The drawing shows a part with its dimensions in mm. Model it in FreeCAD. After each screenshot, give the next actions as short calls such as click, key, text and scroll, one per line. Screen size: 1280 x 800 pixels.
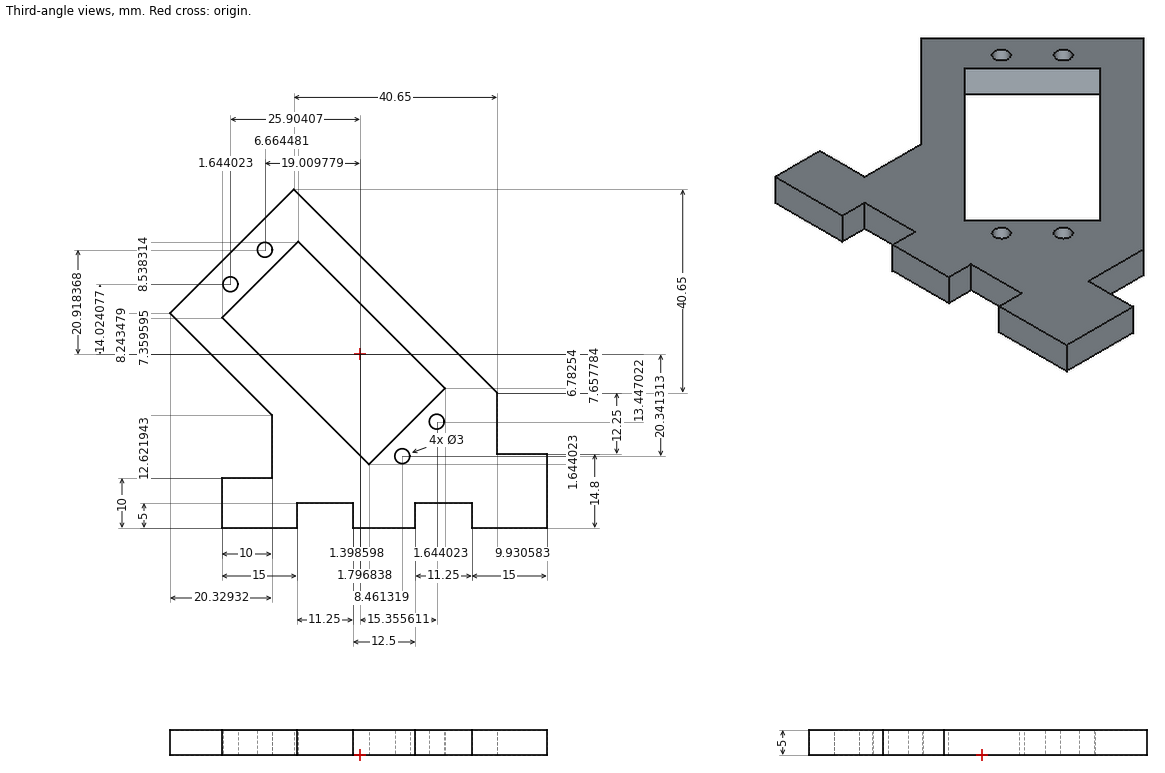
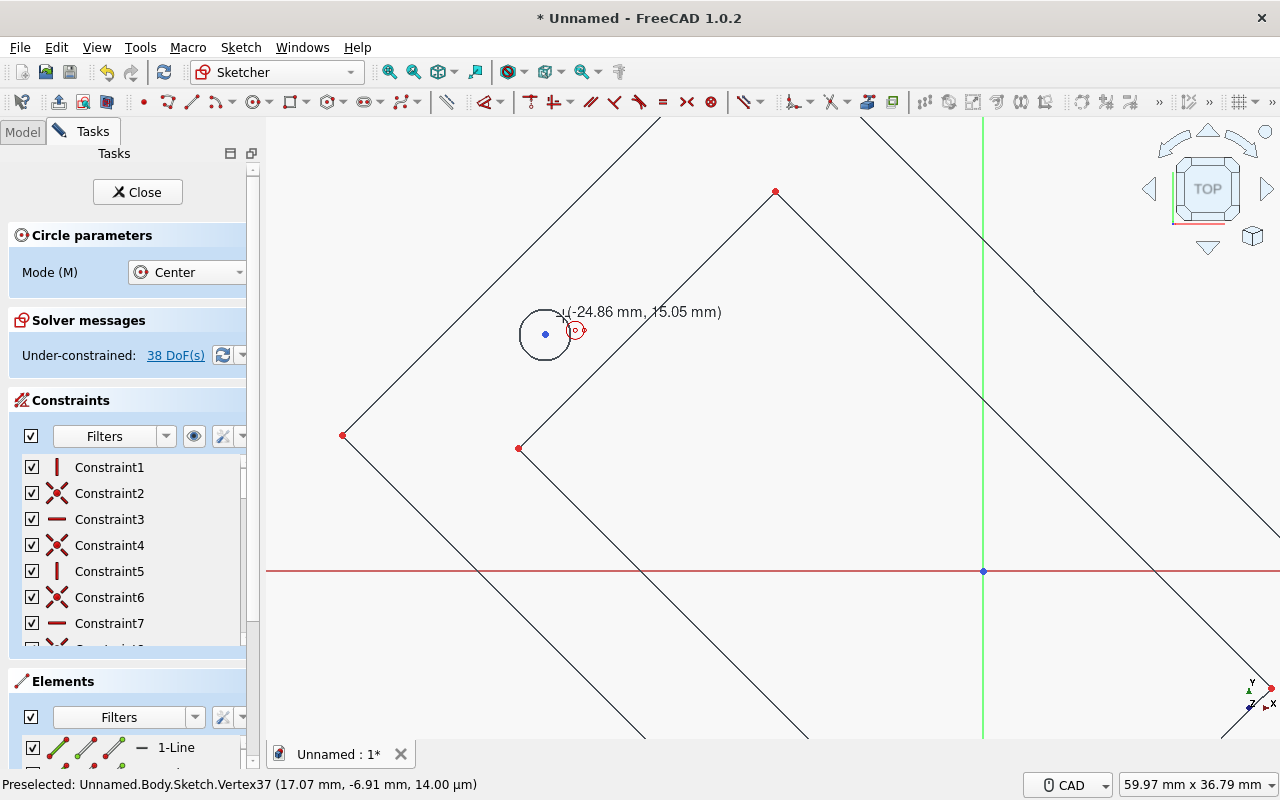
click(662, 218)
click(680, 200)
key(Escape)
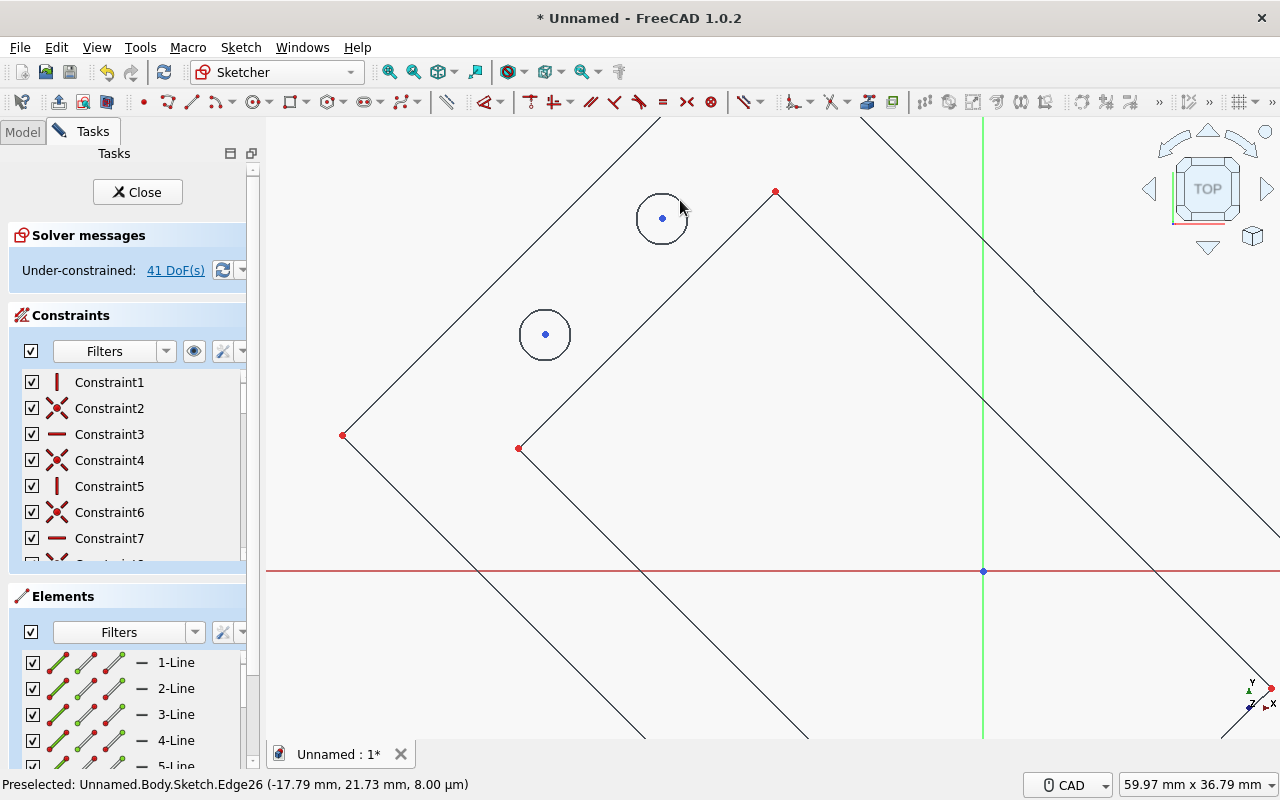
scroll(545, 336, down, 5)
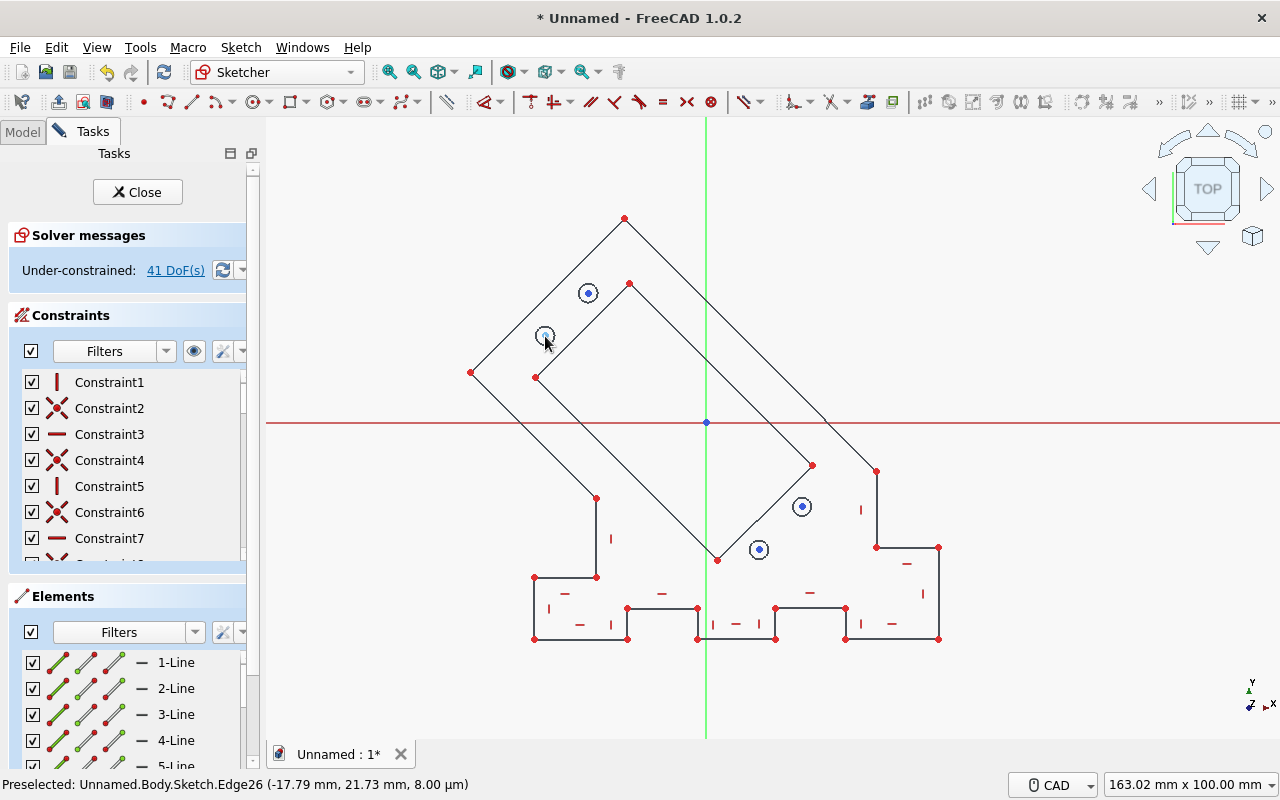
scroll(766, 543, up, 2)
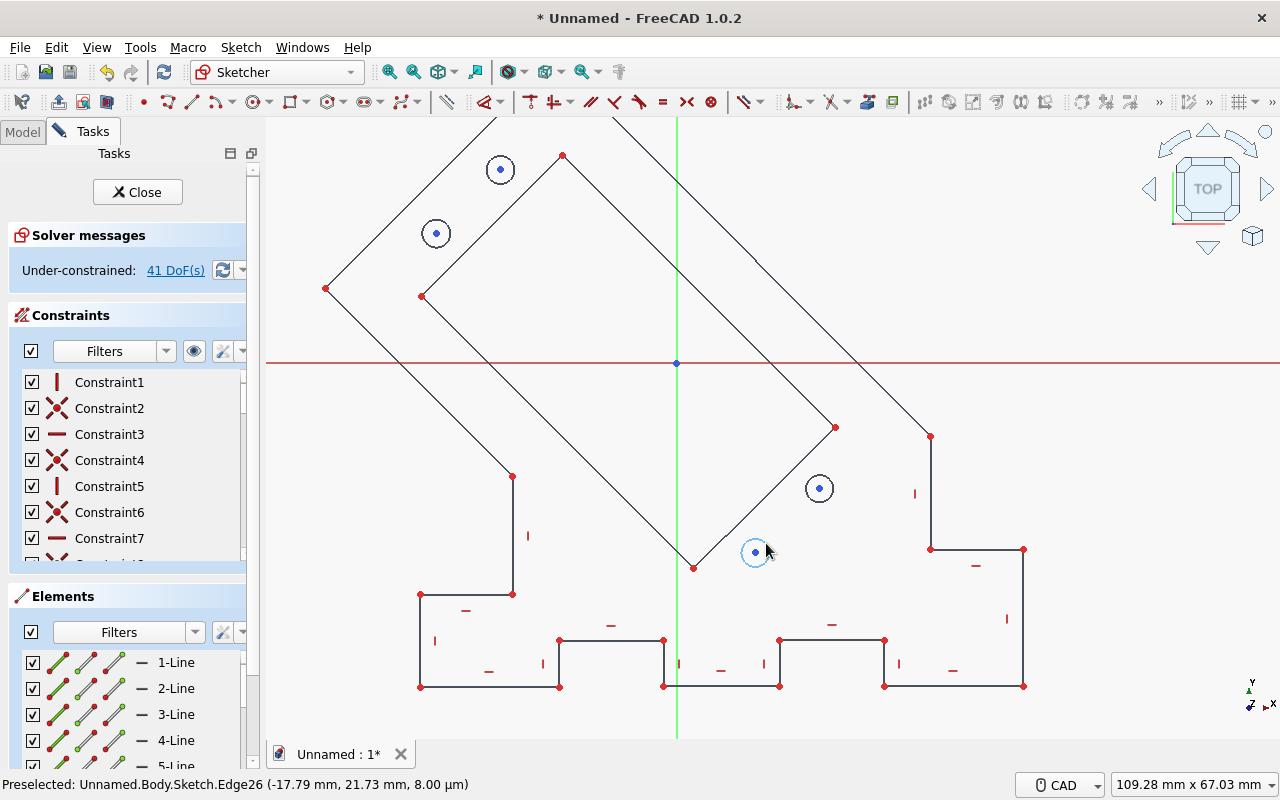
click(765, 543)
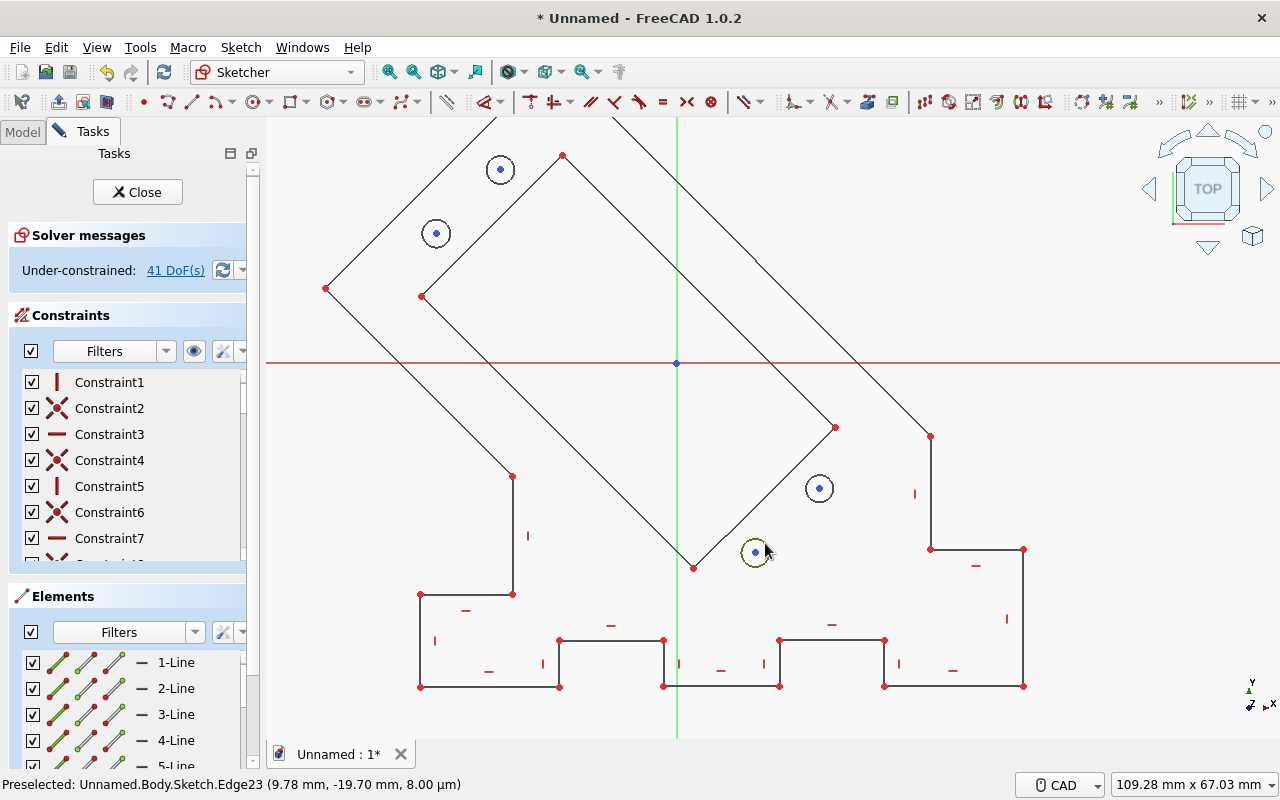
click(829, 479)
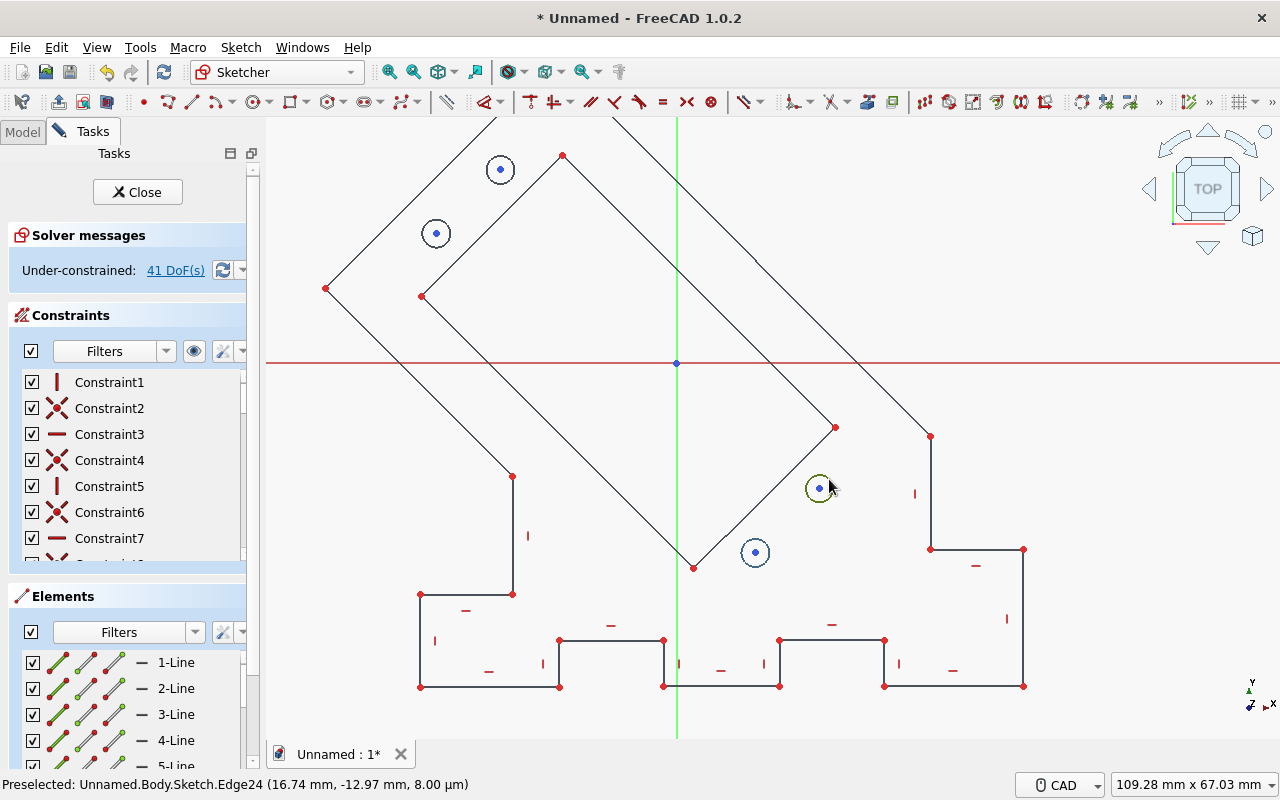
click(446, 224)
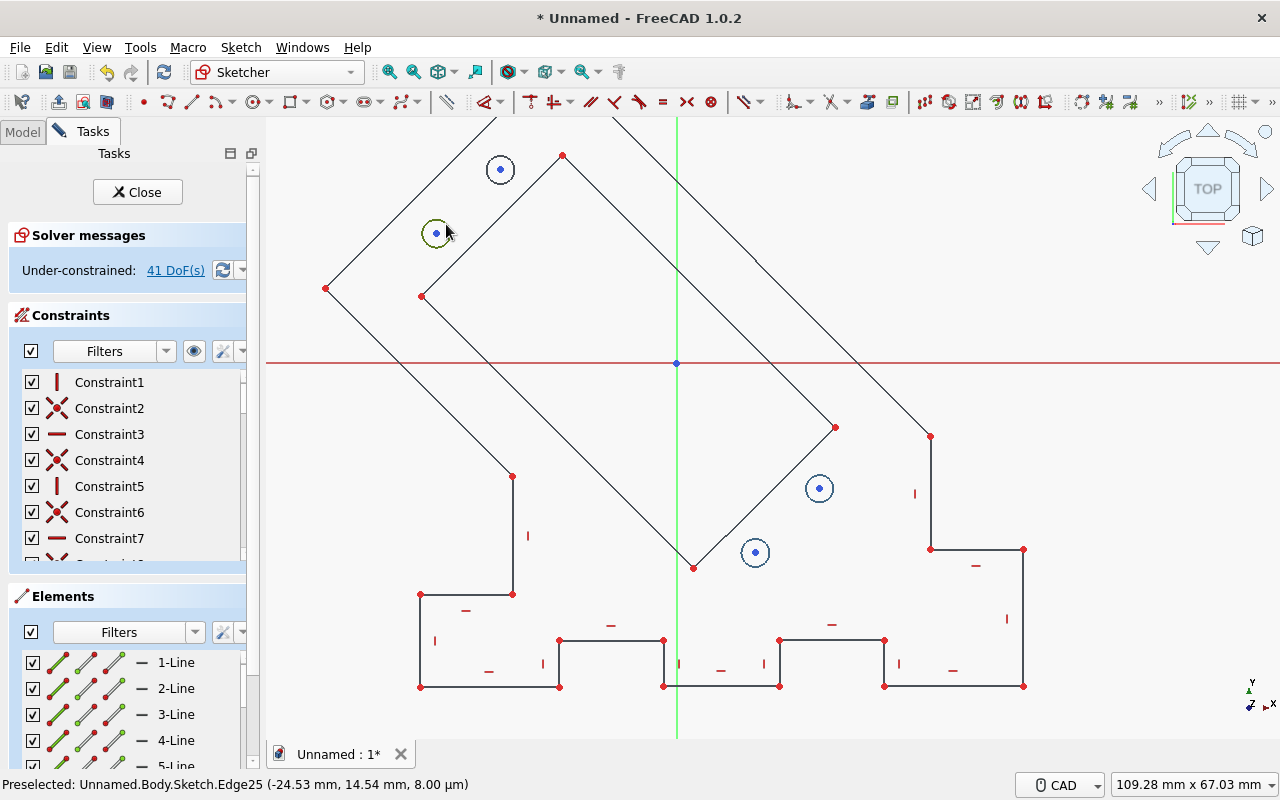
click(510, 160)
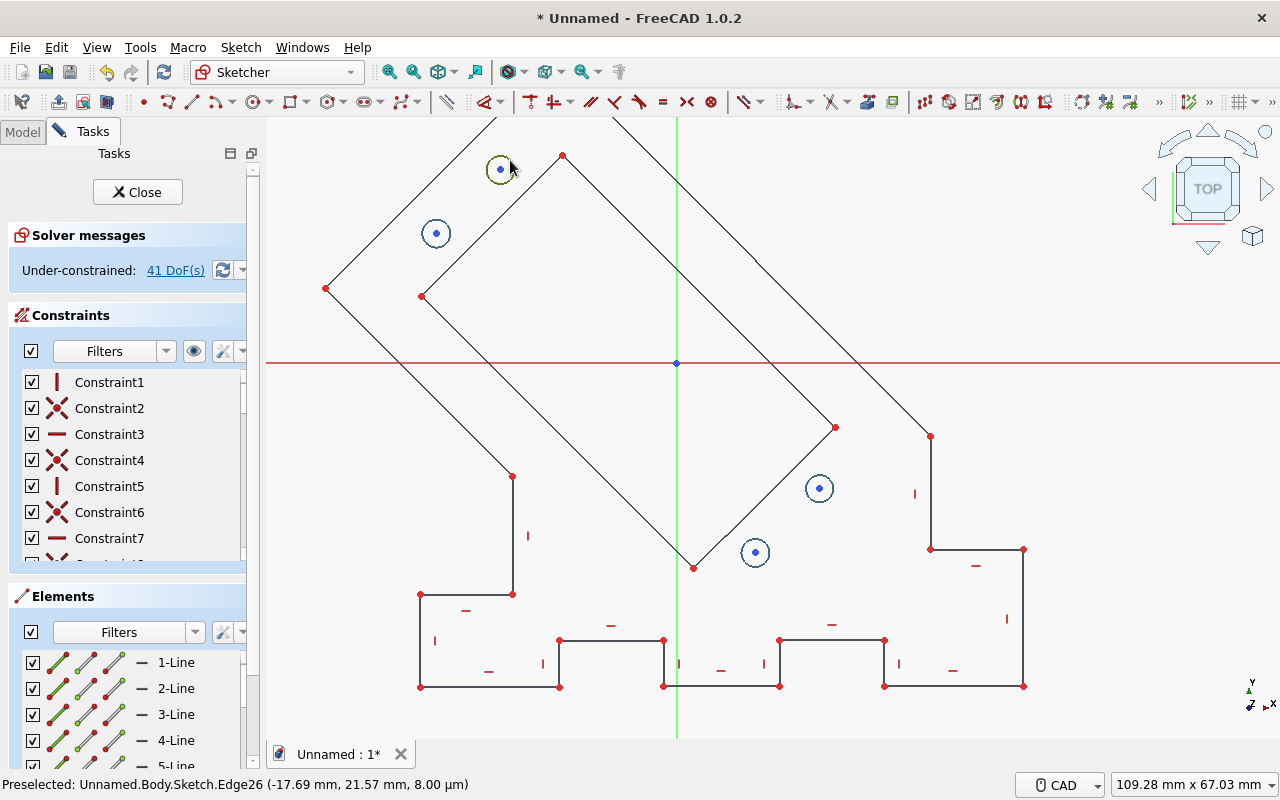
click(664, 102)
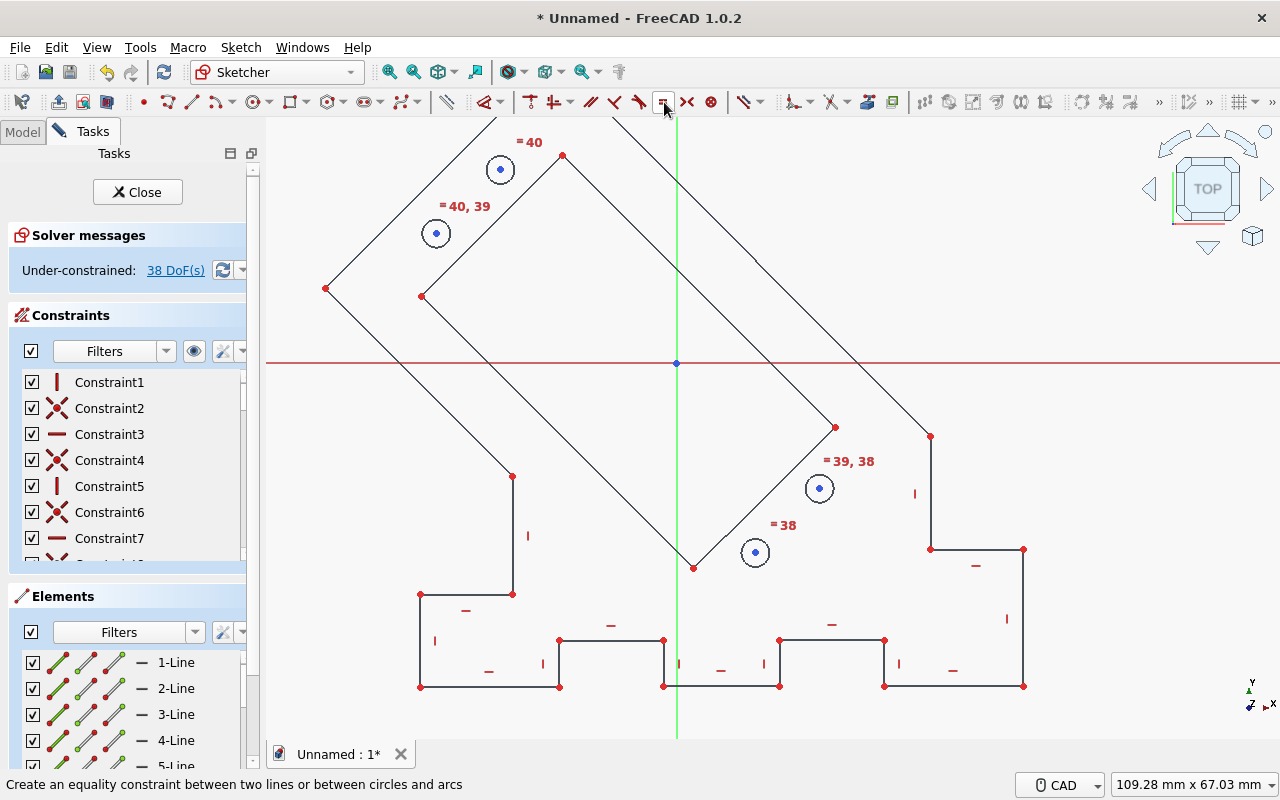
click(484, 102)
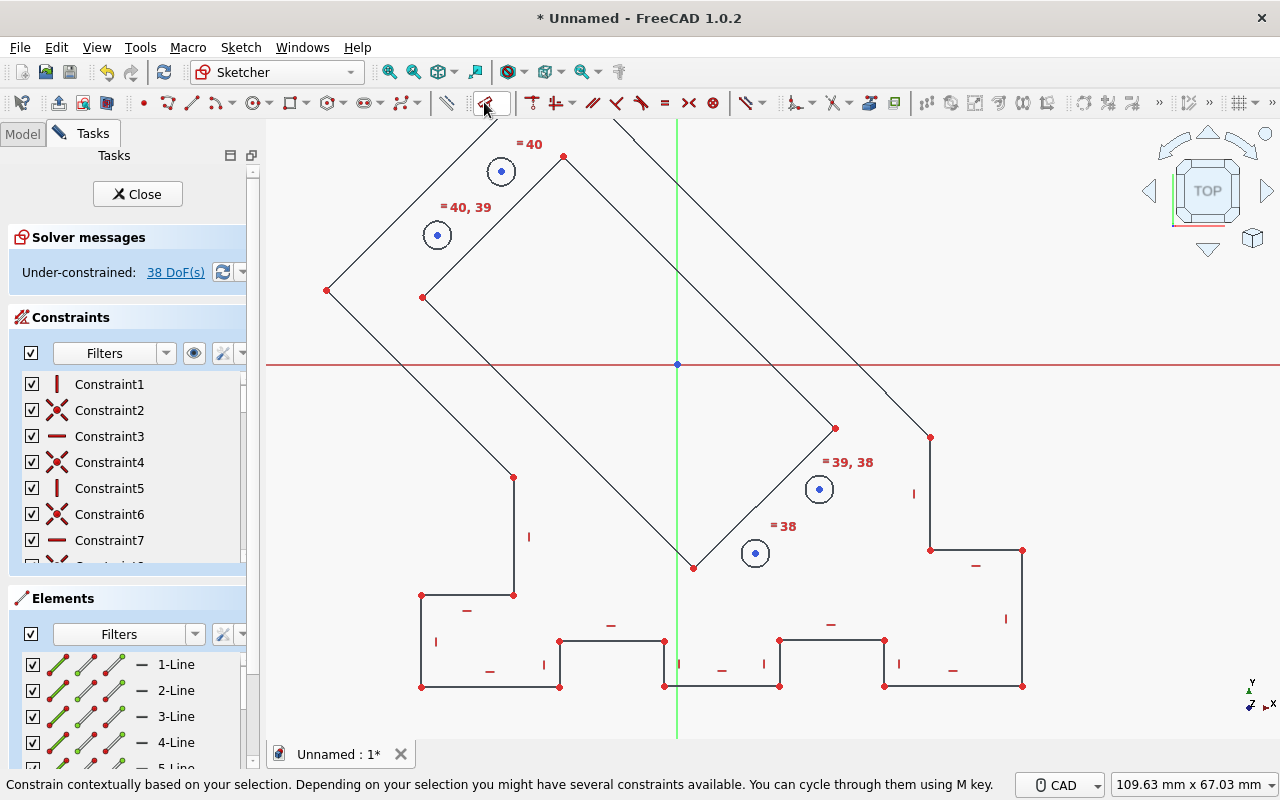
scroll(765, 544, up, 2)